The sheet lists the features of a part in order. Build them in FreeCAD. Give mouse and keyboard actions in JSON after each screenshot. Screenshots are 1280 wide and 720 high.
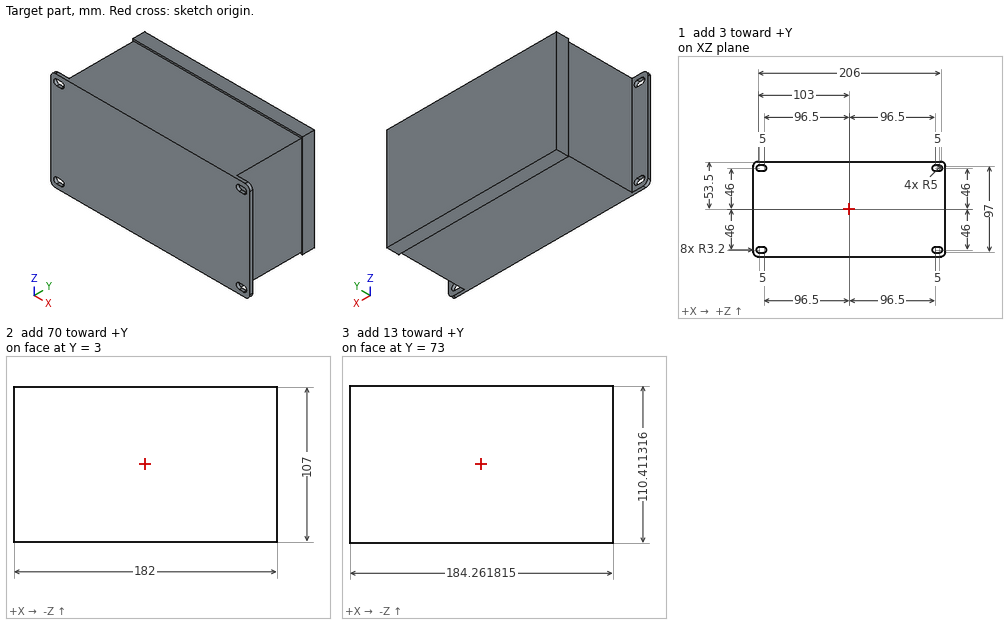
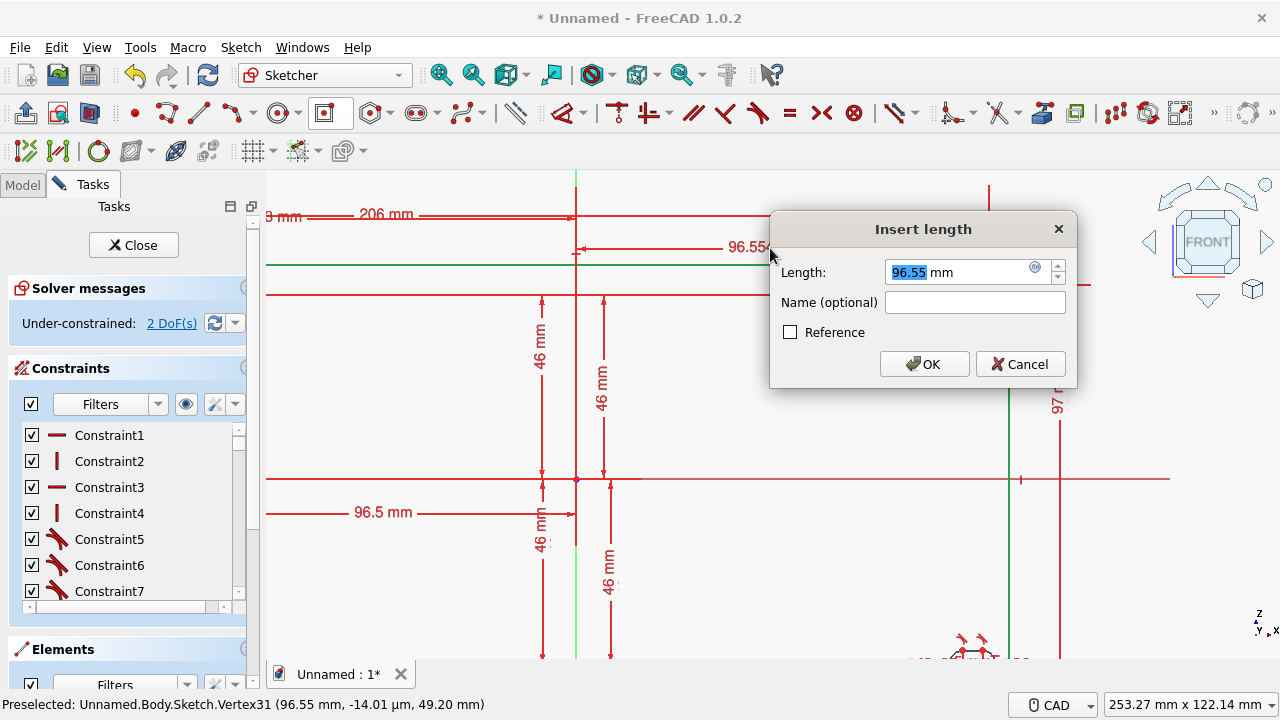
{"action": "type", "text": "96.5"}
{"action": "key", "text": "Return"}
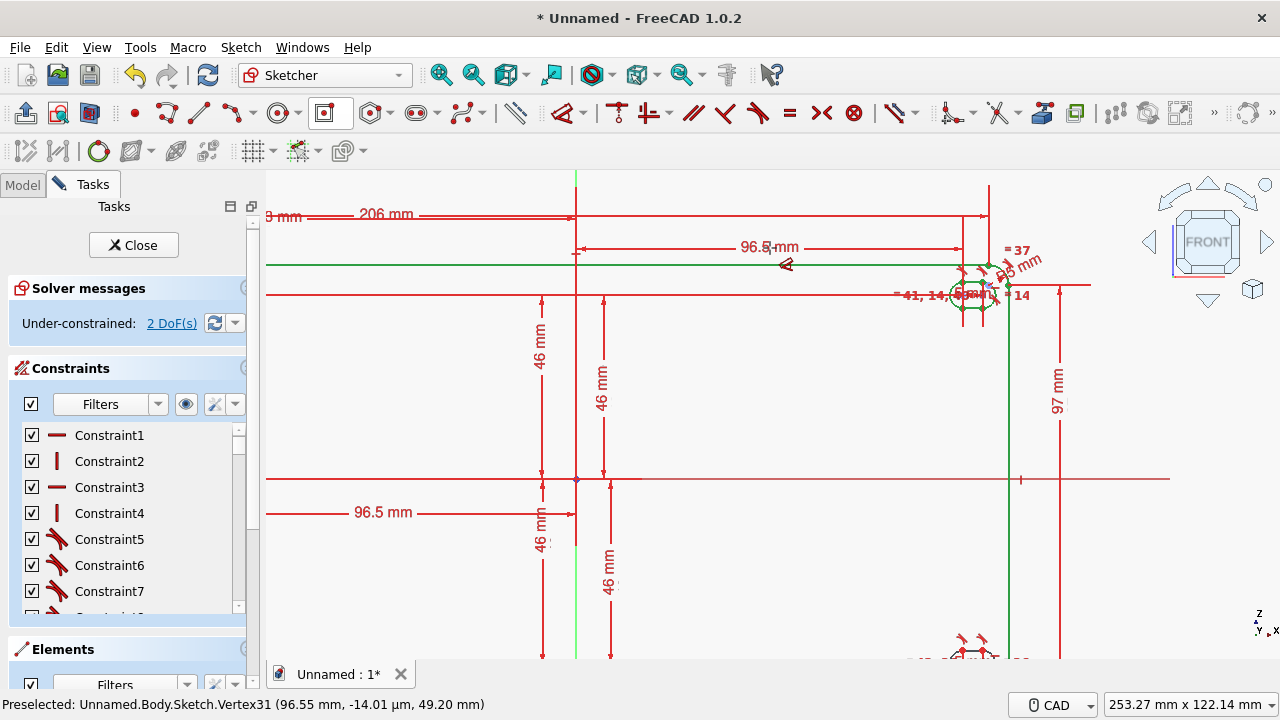
{"action": "scroll", "coordinate": [965, 282], "scroll_direction": "down", "scroll_amount": 2}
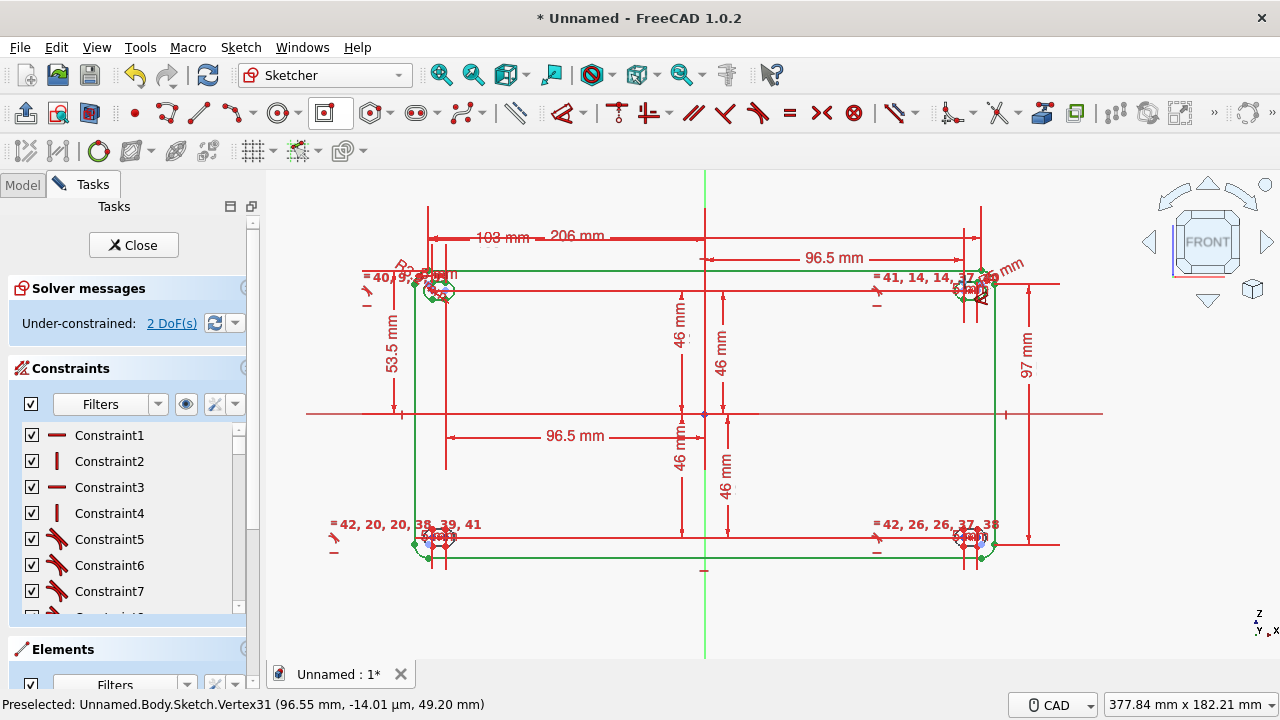
{"action": "scroll", "coordinate": [446, 546], "scroll_direction": "up", "scroll_amount": 2}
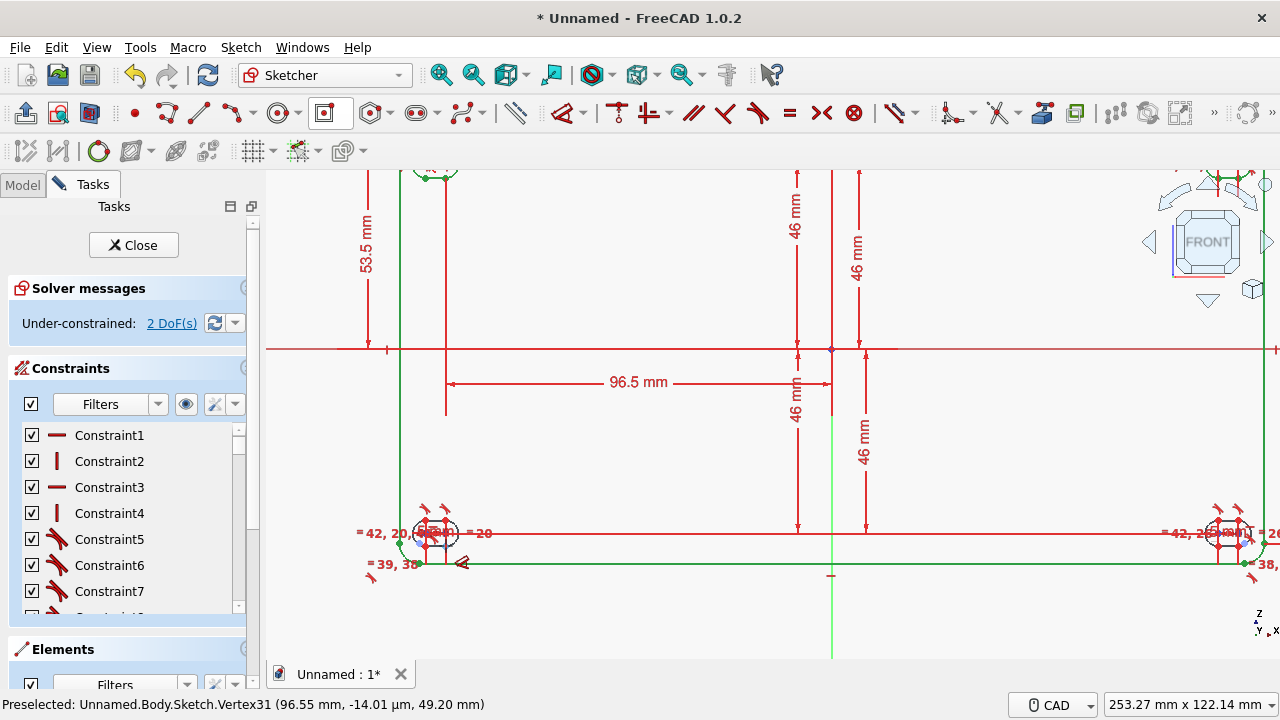
{"action": "left_click", "coordinate": [446, 546]}
{"action": "left_click", "coordinate": [639, 580]}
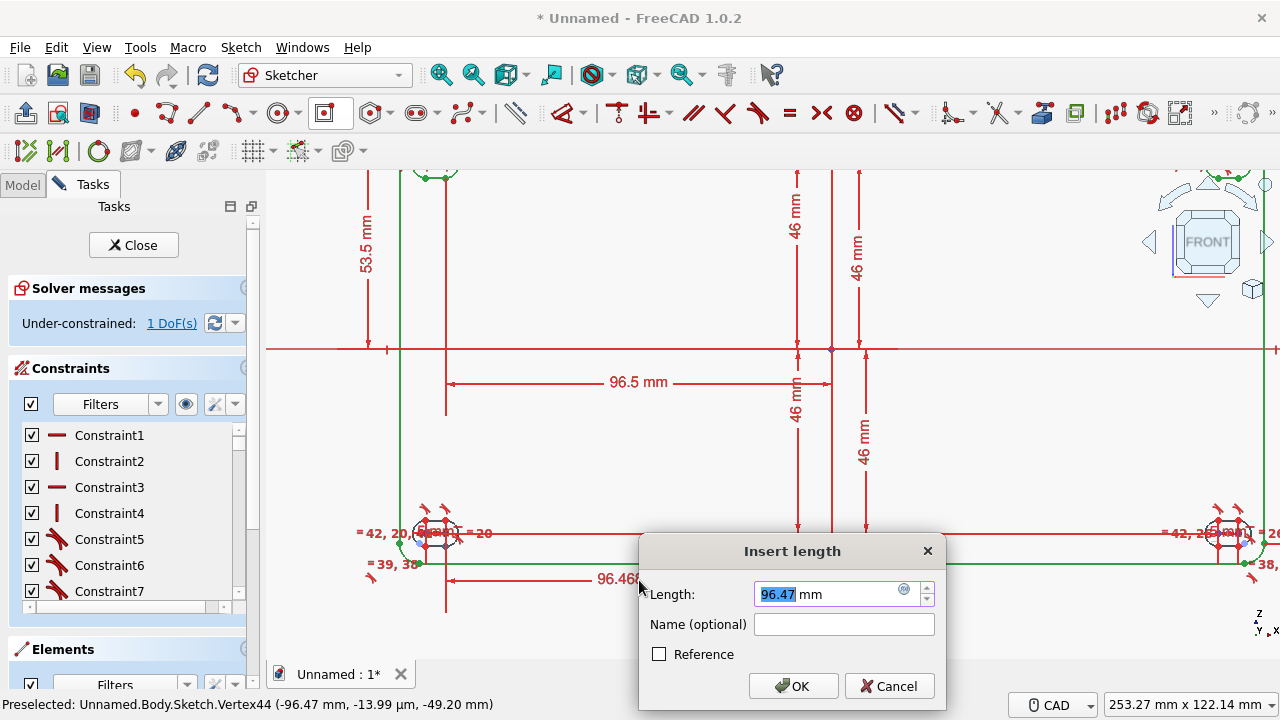
{"action": "type", "text": "96.5"}
{"action": "key", "text": "Return"}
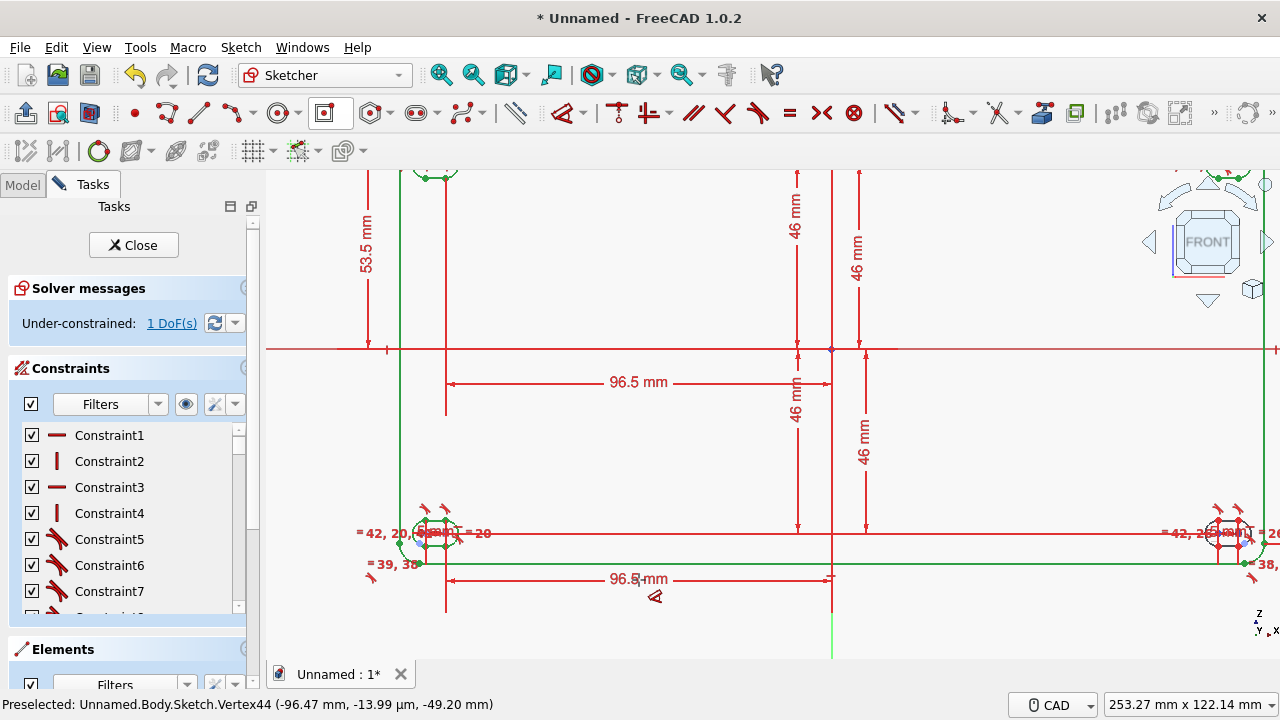
{"action": "scroll", "coordinate": [445, 547], "scroll_direction": "down", "scroll_amount": 2}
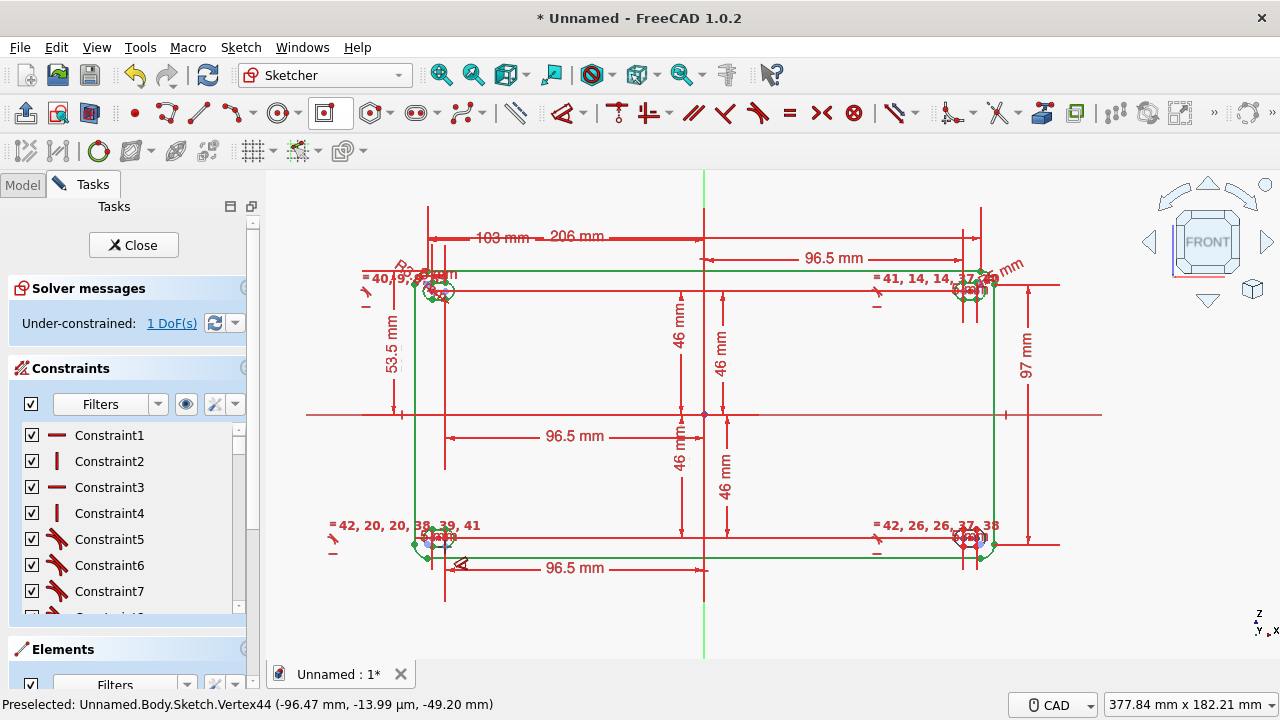
{"action": "scroll", "coordinate": [963, 530], "scroll_direction": "up", "scroll_amount": 2}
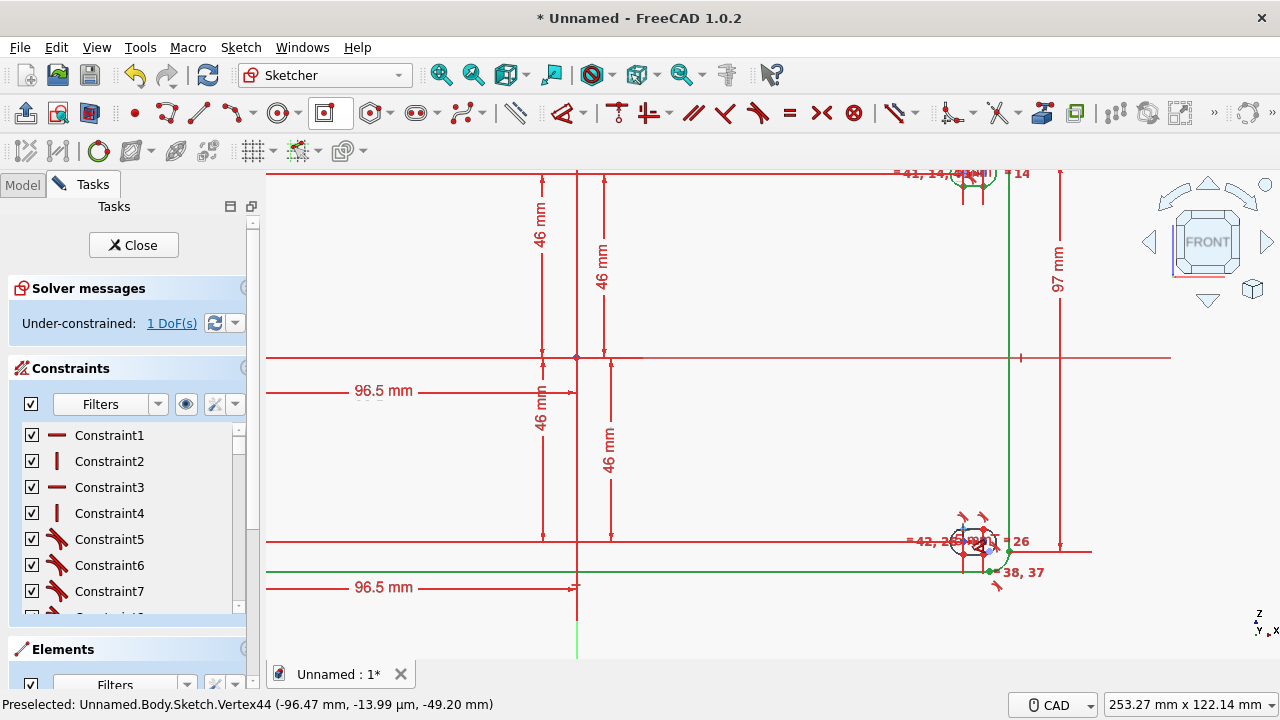
{"action": "left_click", "coordinate": [963, 529]}
{"action": "left_click", "coordinate": [770, 324]}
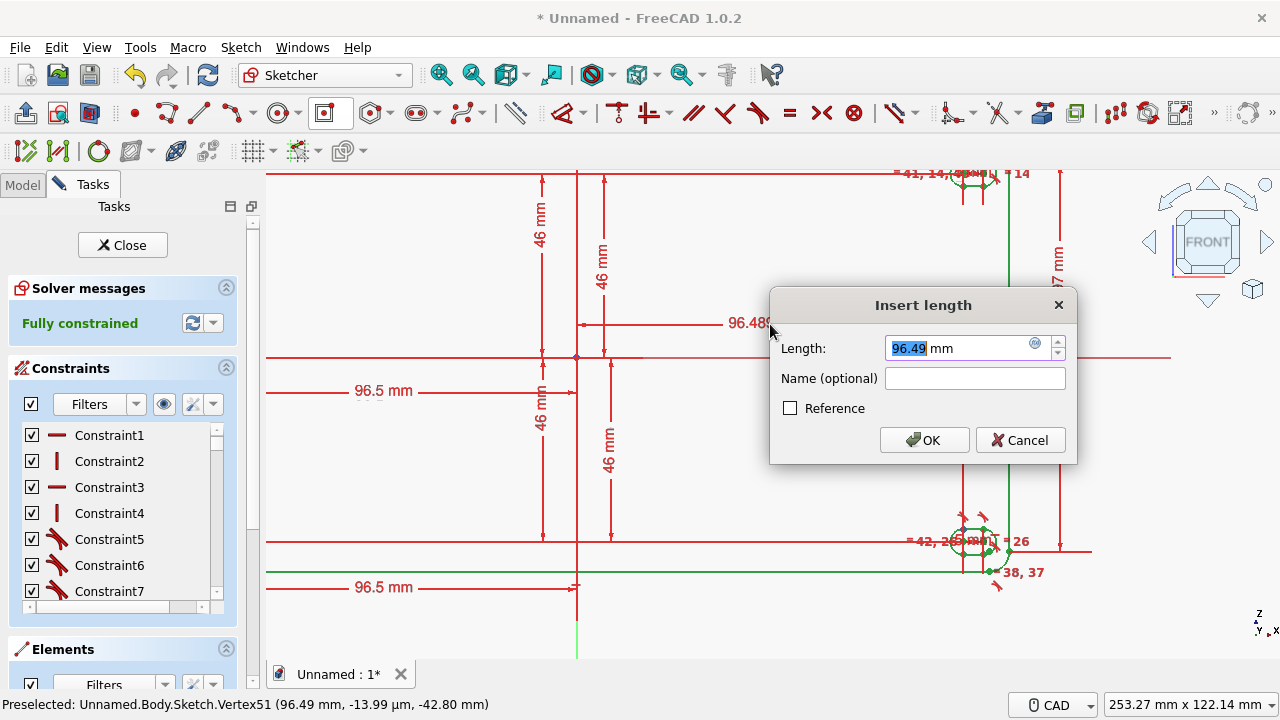
{"action": "type", "text": "96.5"}
{"action": "key", "text": "Return"}
{"action": "key", "text": "Escape"}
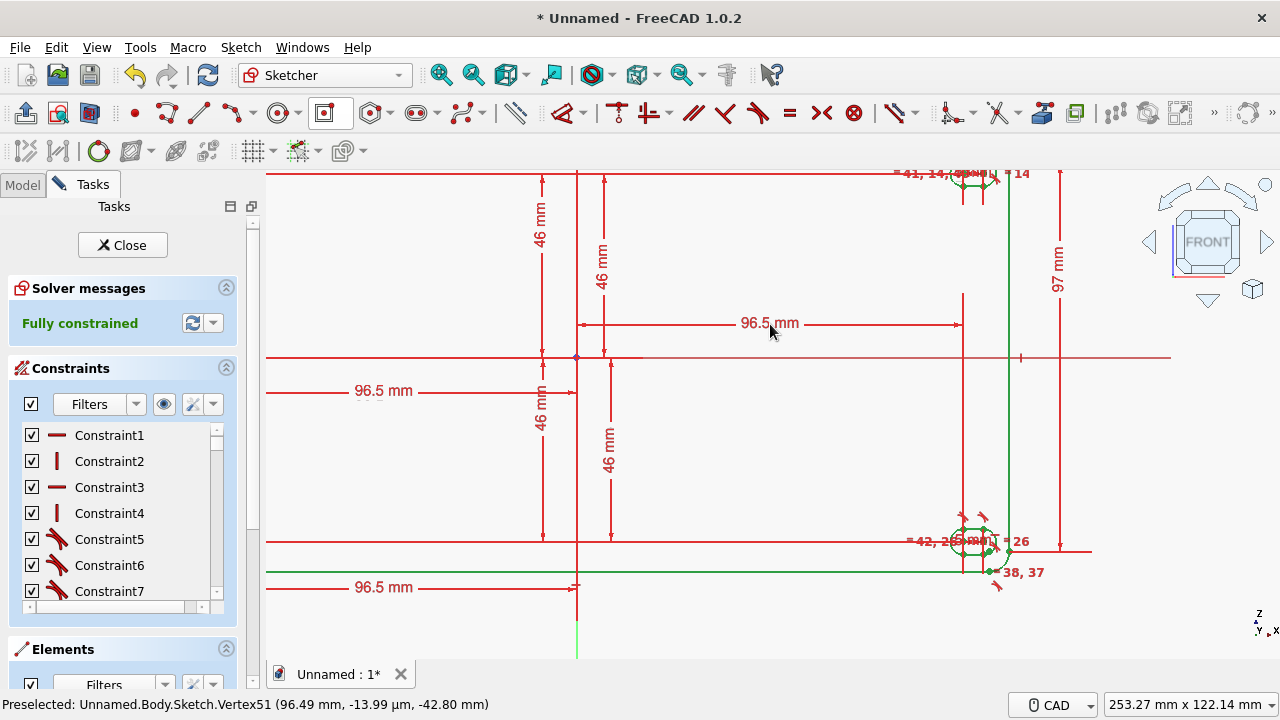
{"action": "left_click", "coordinate": [123, 245]}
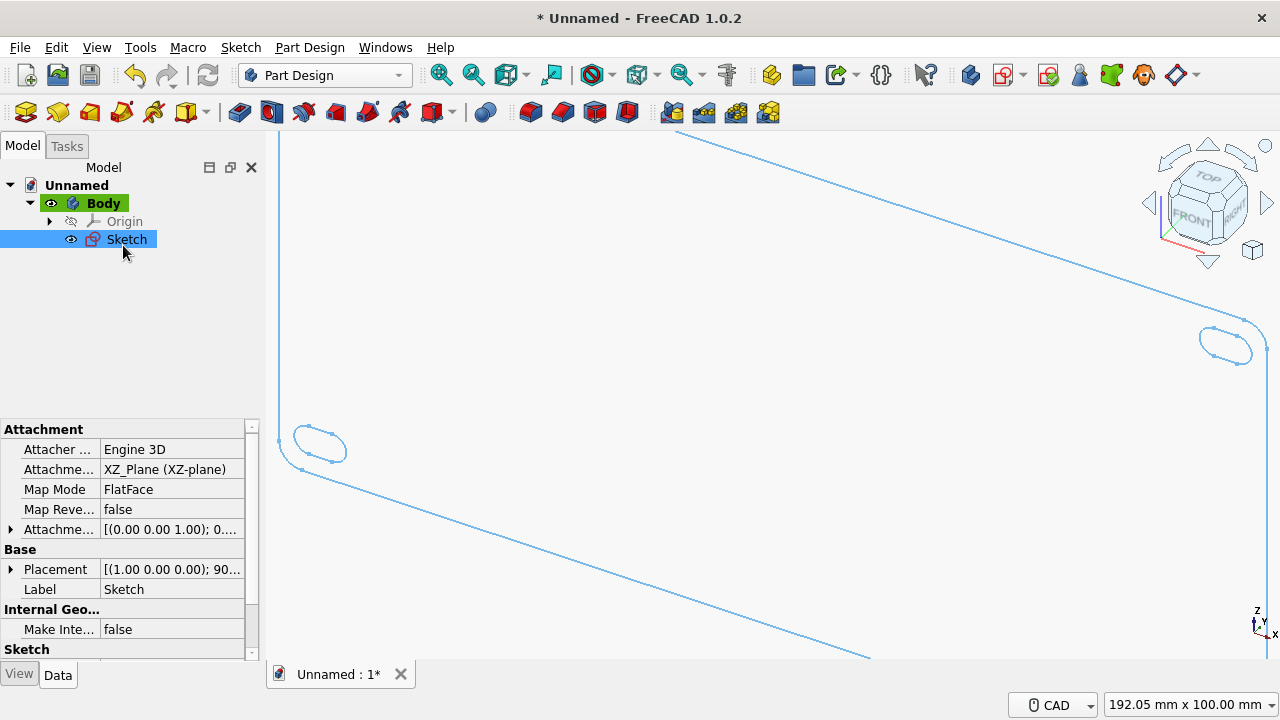
{"action": "left_click", "coordinate": [26, 112]}